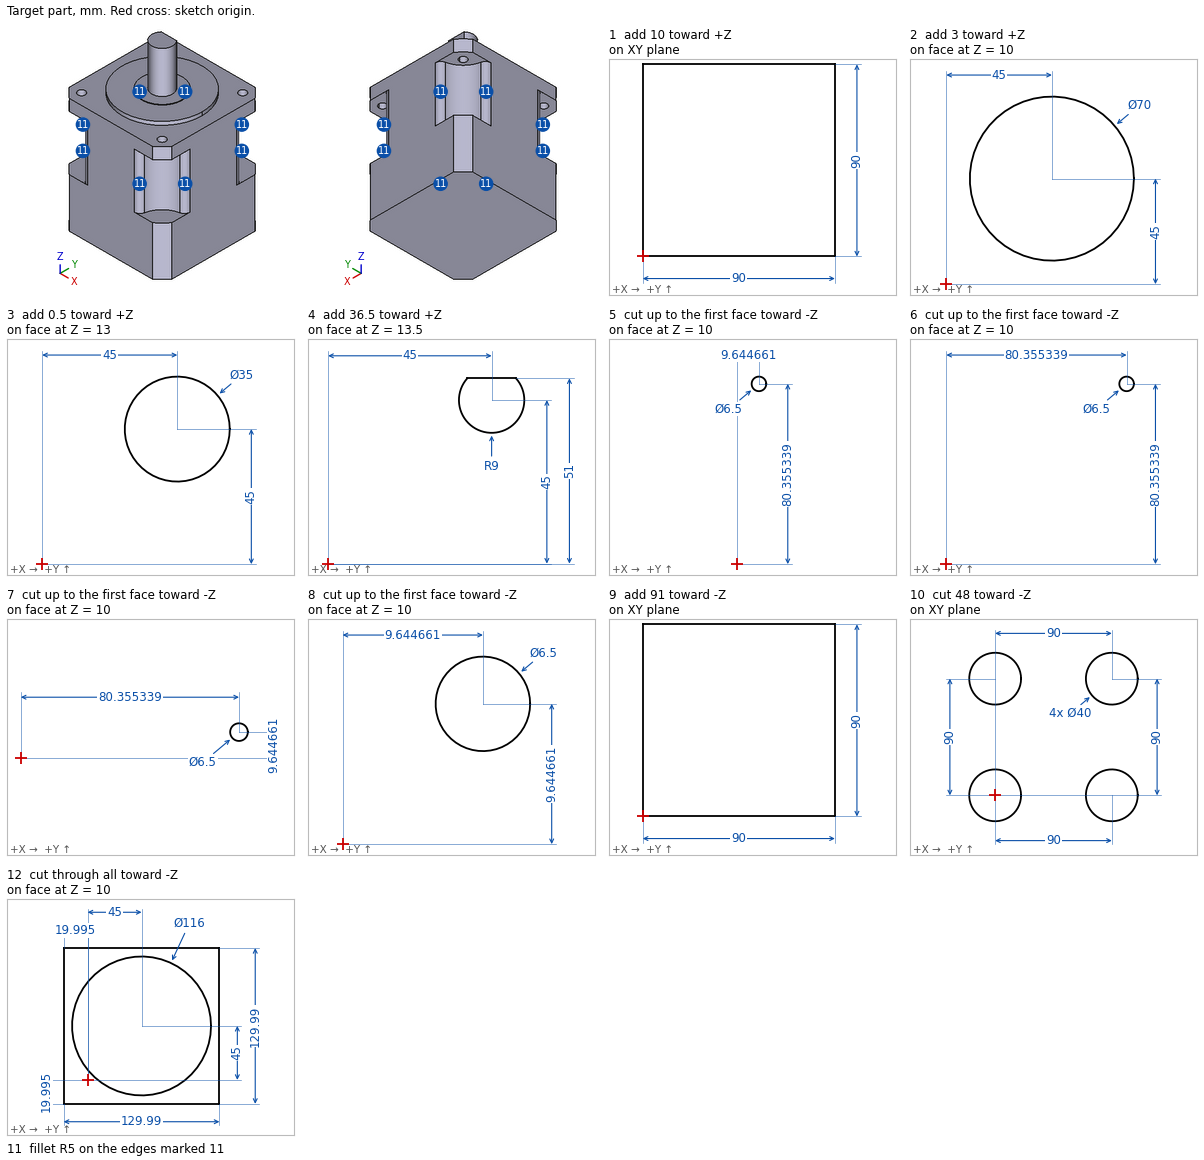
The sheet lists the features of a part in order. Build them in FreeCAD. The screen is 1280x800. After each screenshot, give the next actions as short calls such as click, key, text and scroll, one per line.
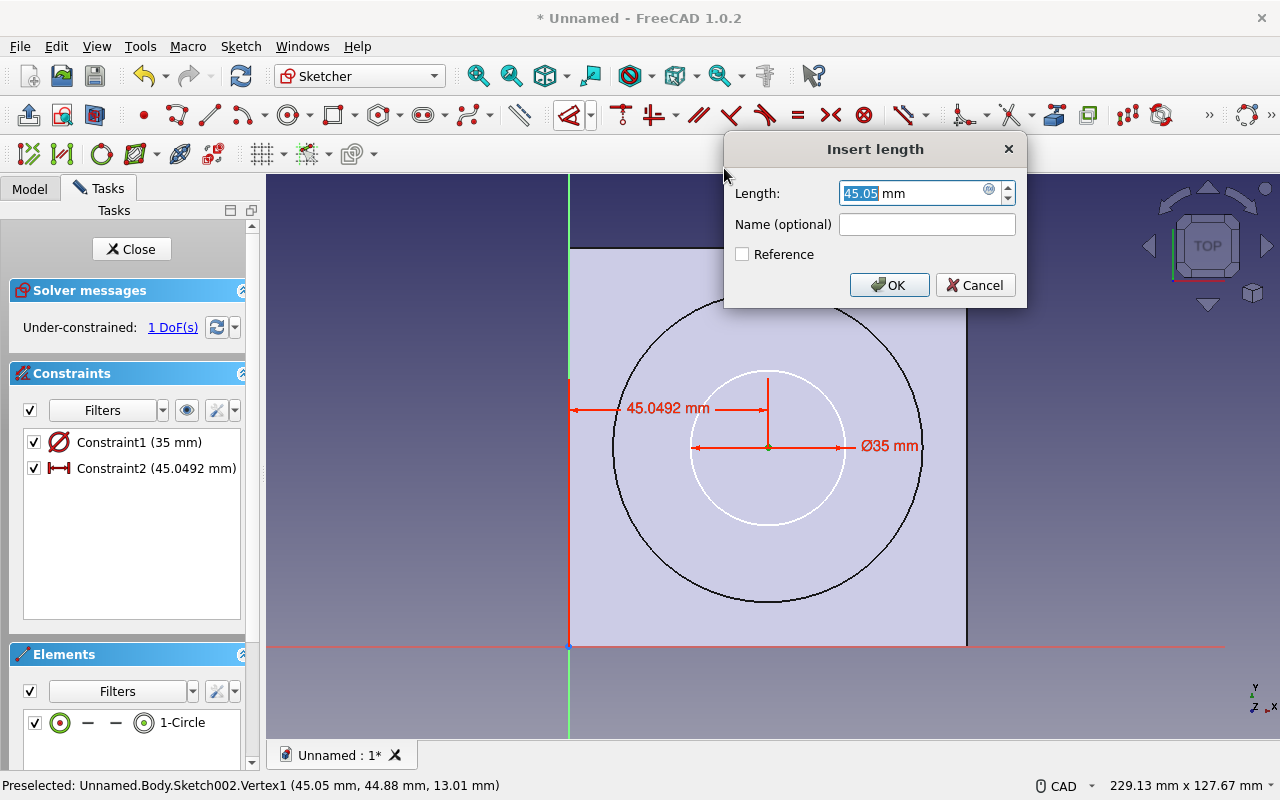
text(45)
key(Return)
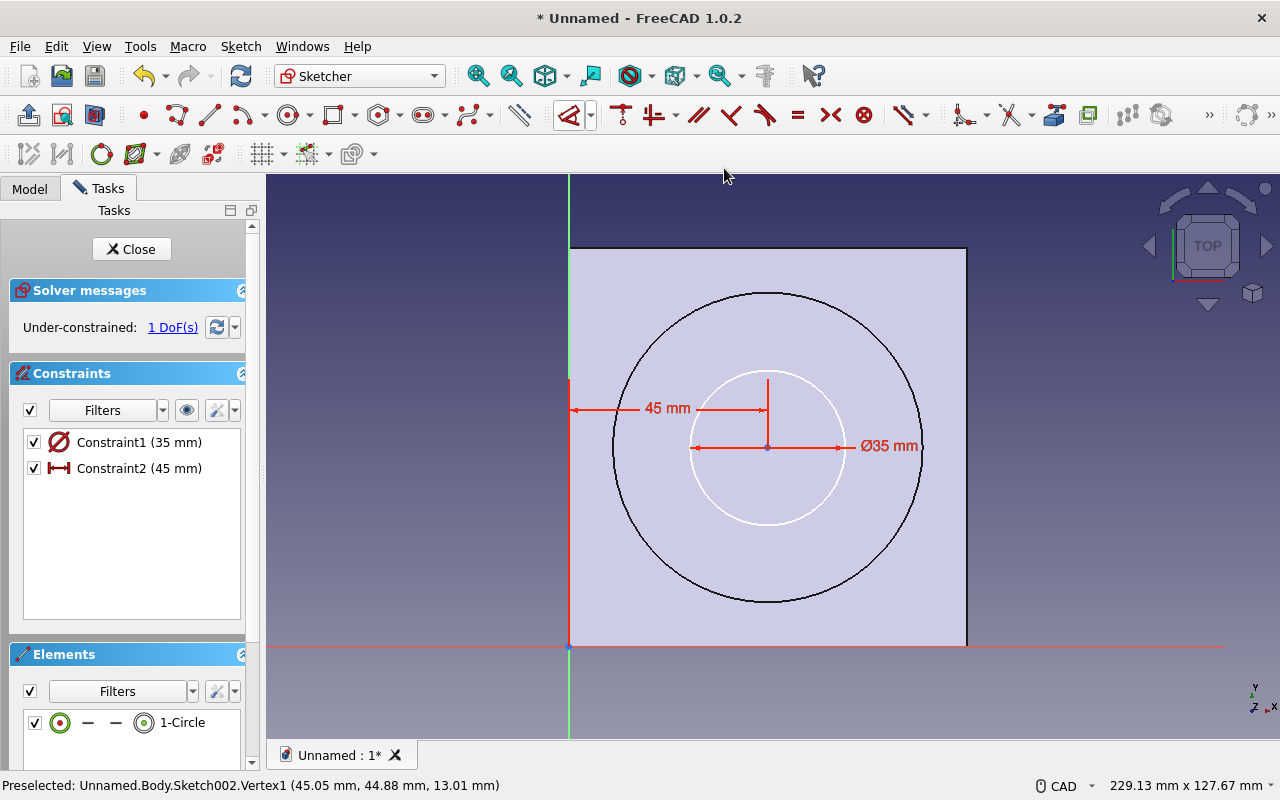
click(768, 448)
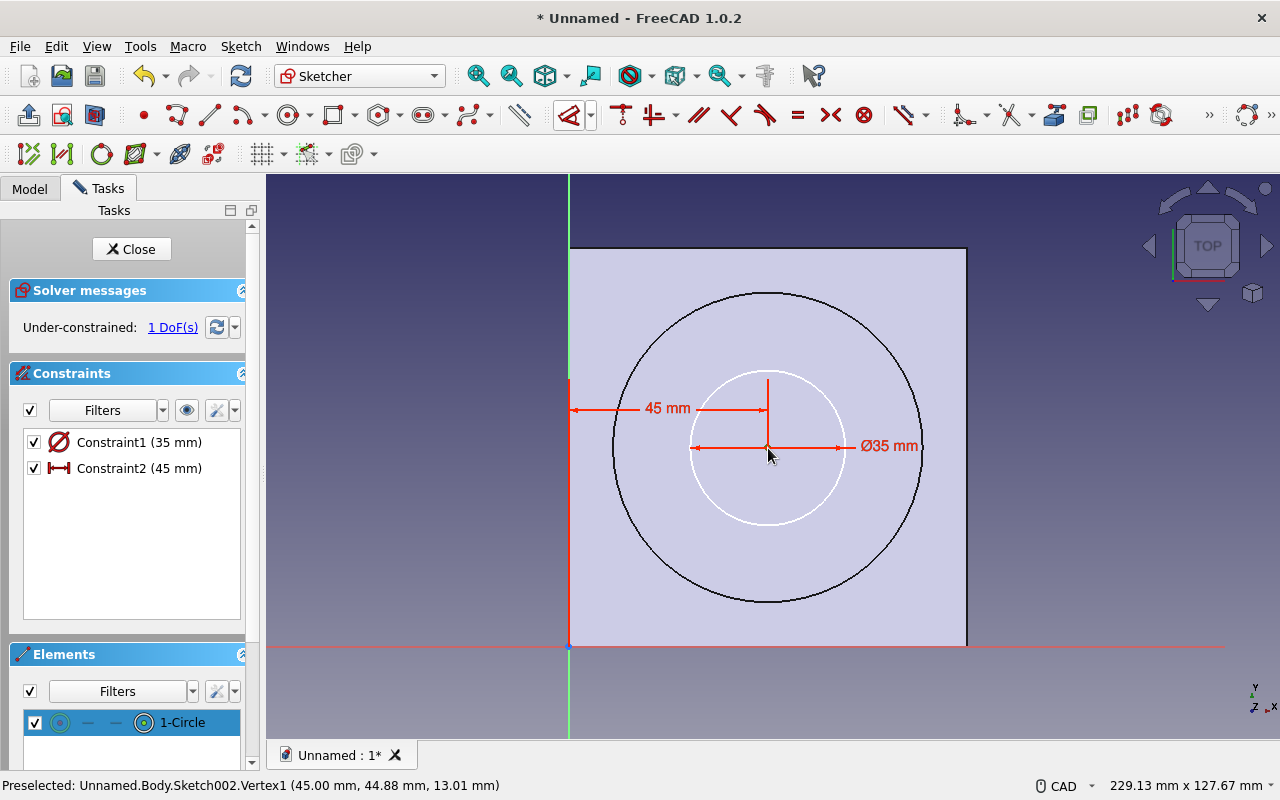
key(i)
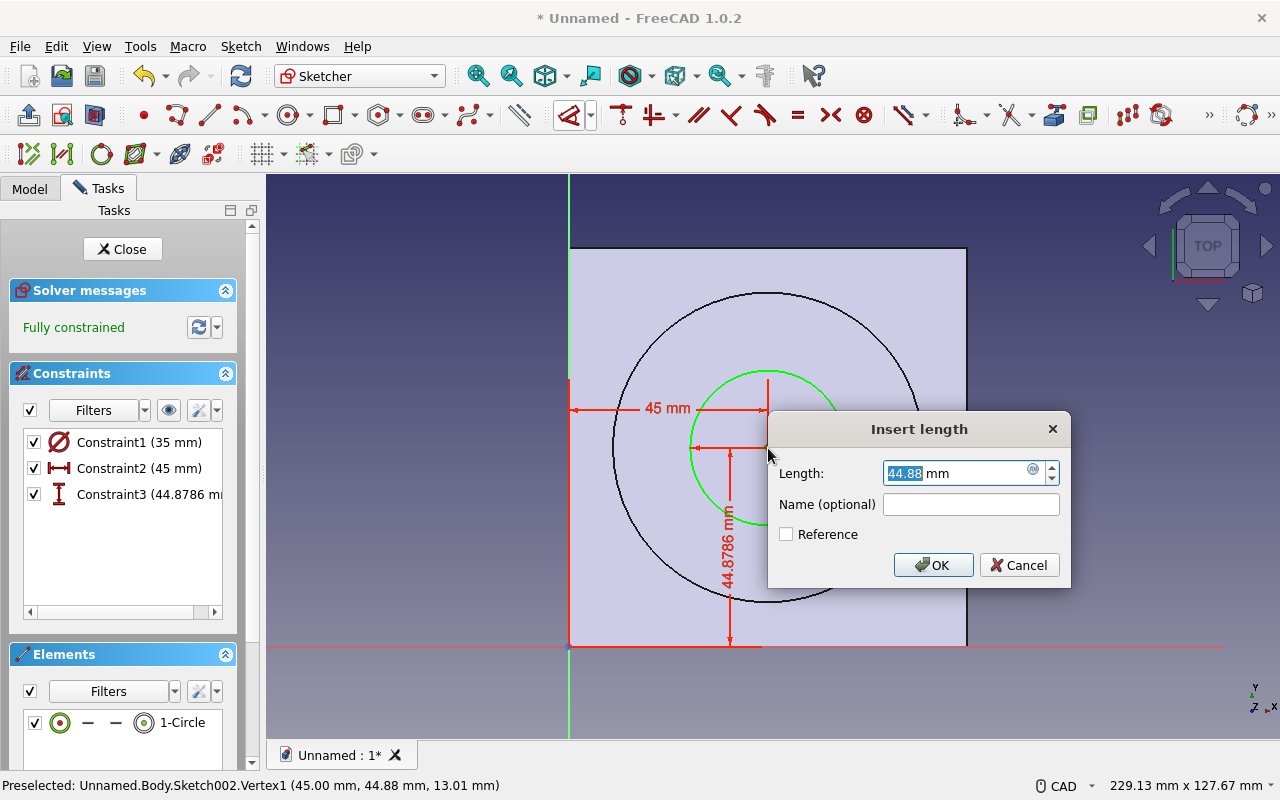
text(45)
key(Return)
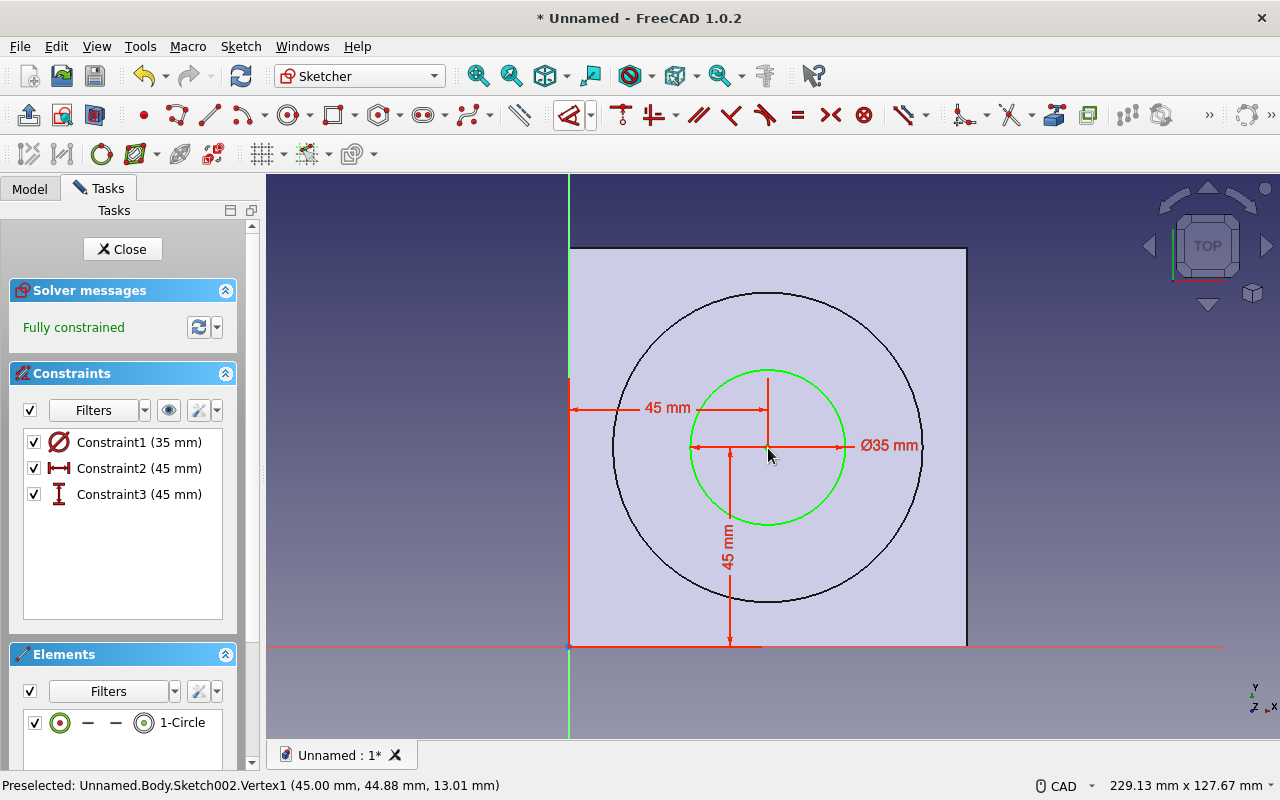
click(123, 249)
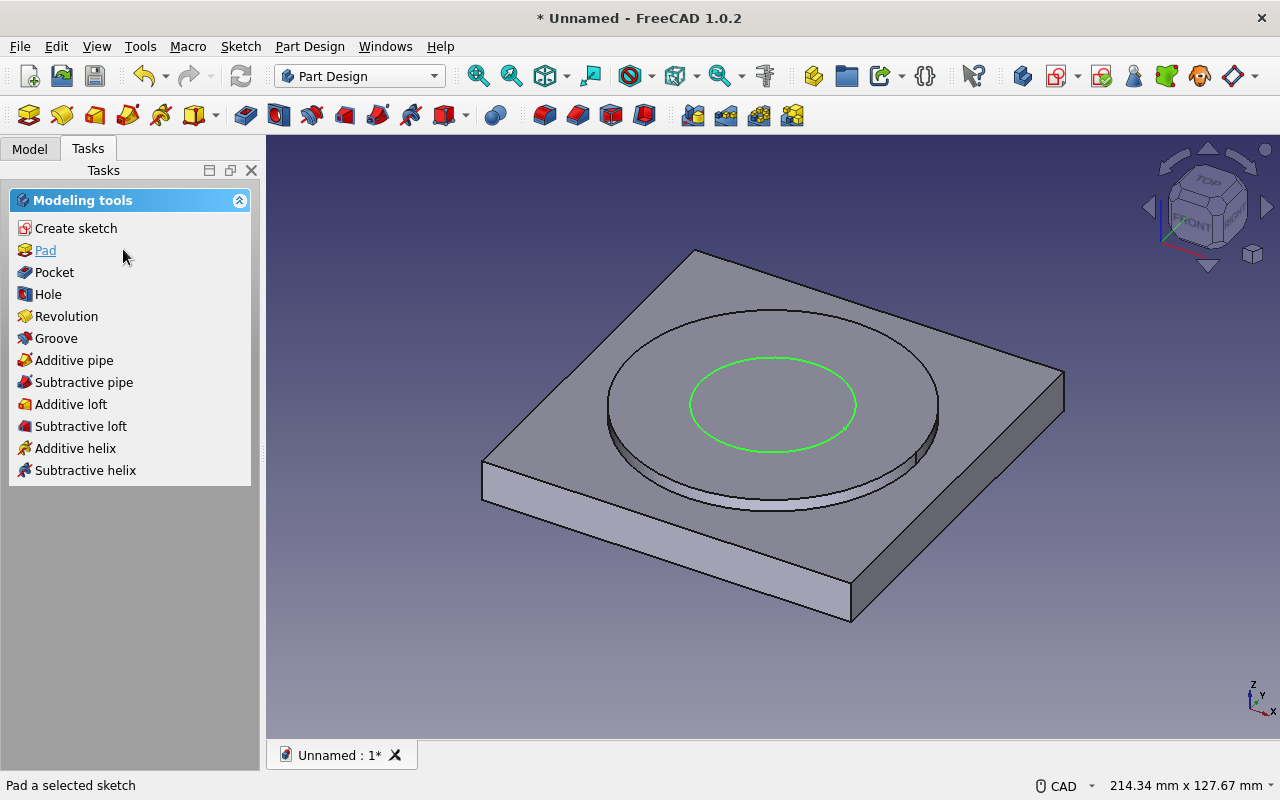
click(29, 116)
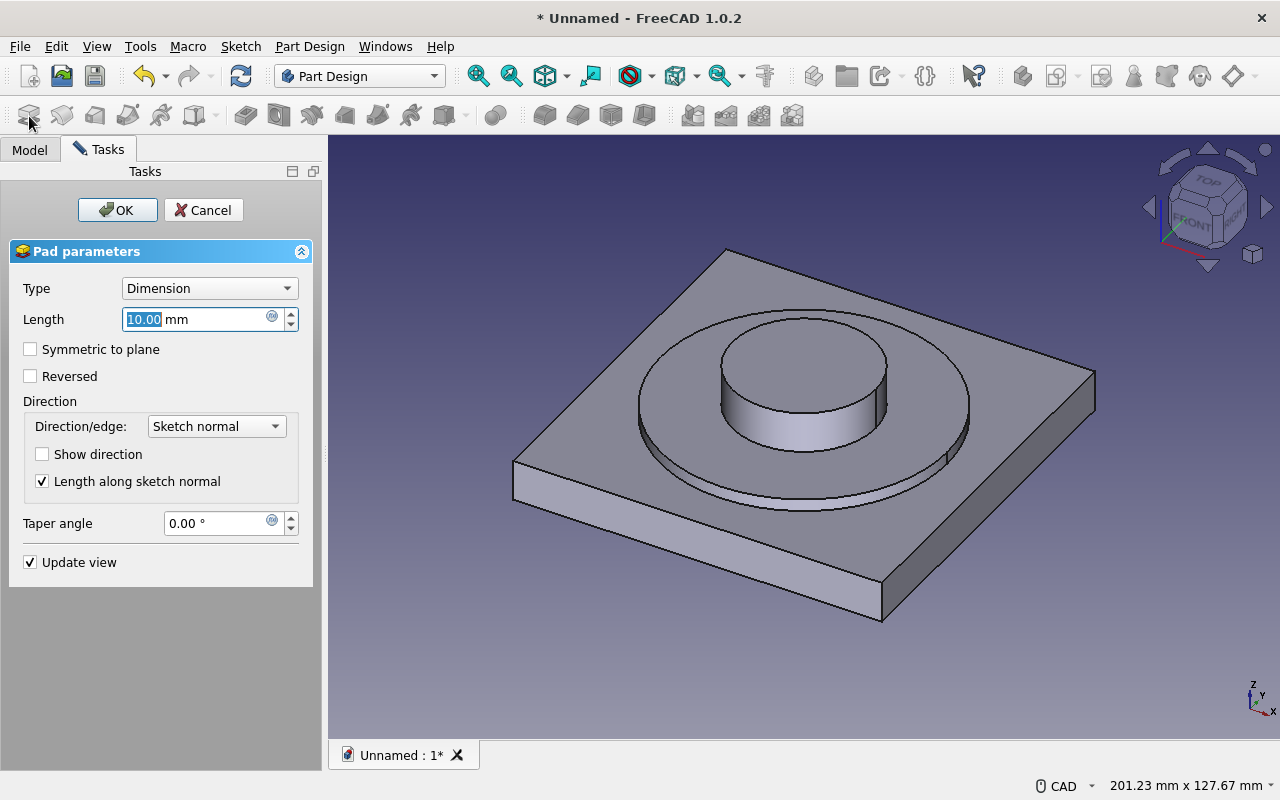
text(0.5)
key(Tab)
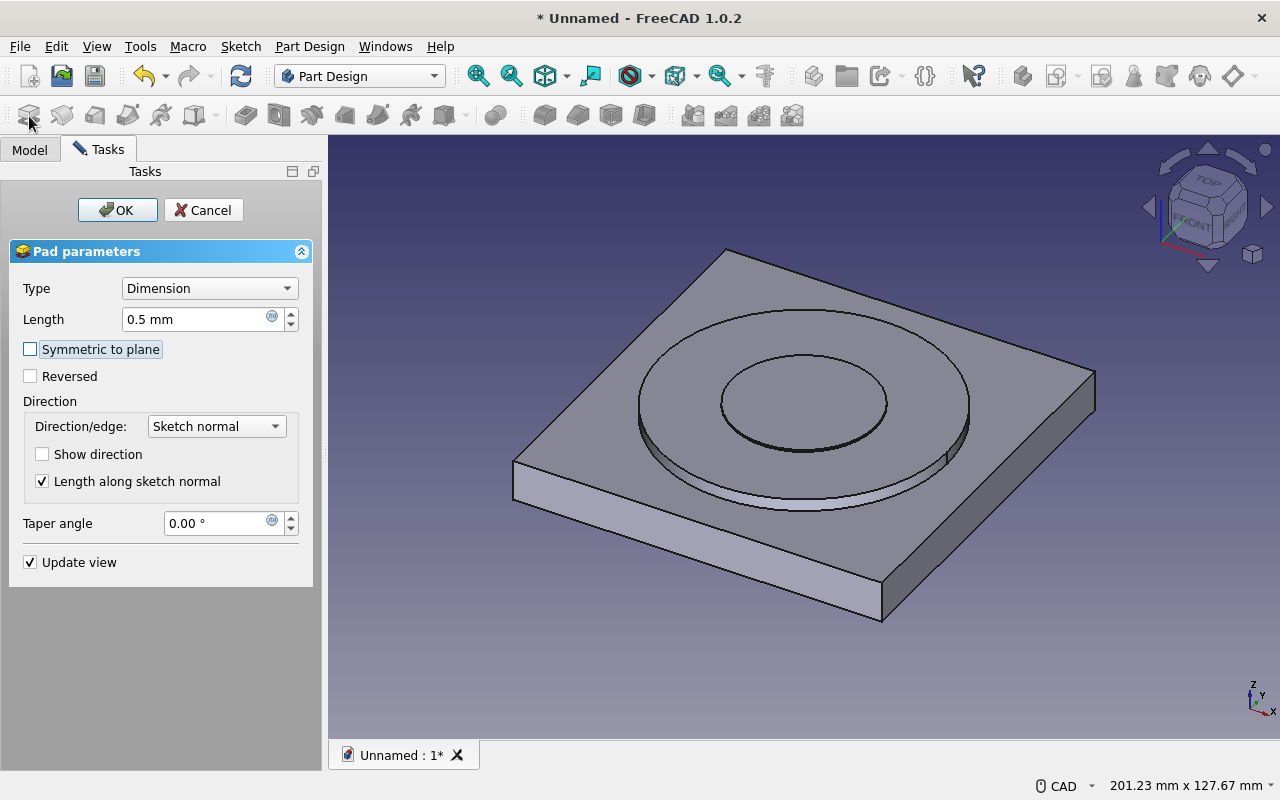
click(118, 210)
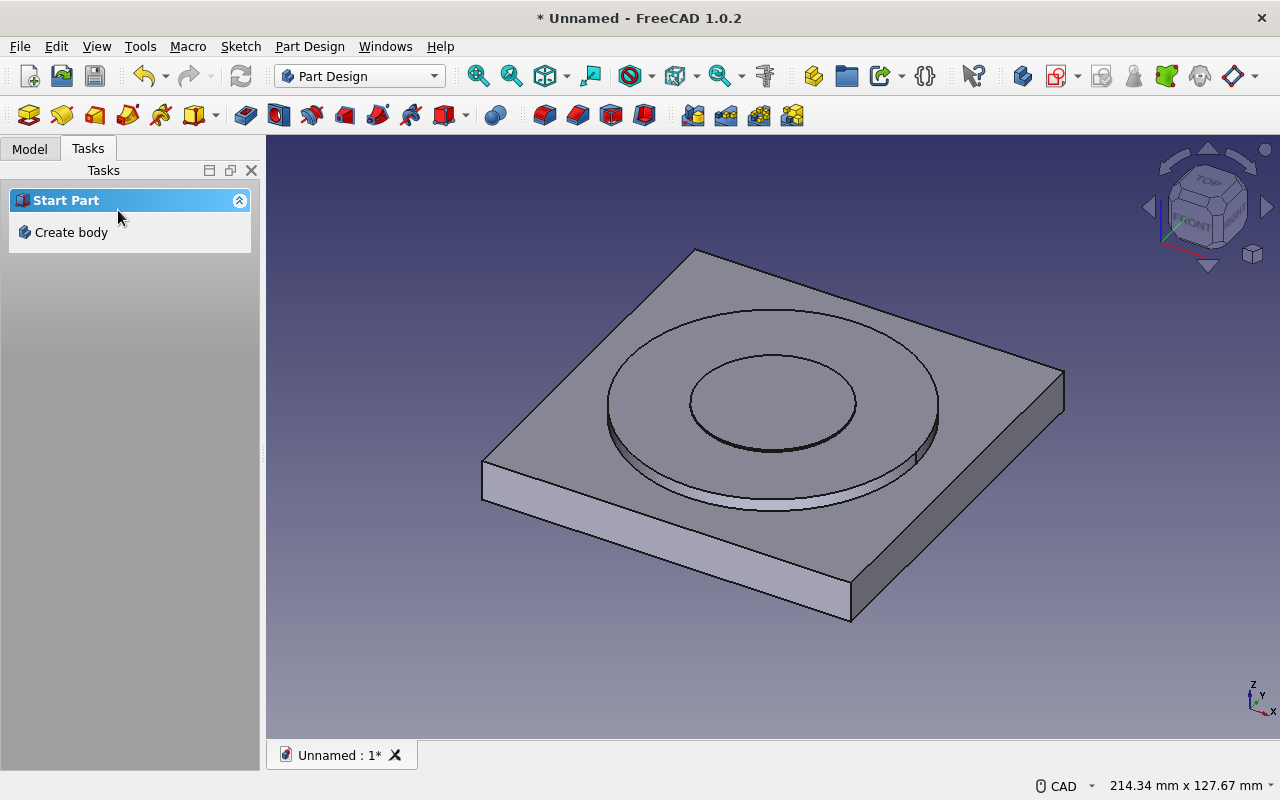
click(773, 402)